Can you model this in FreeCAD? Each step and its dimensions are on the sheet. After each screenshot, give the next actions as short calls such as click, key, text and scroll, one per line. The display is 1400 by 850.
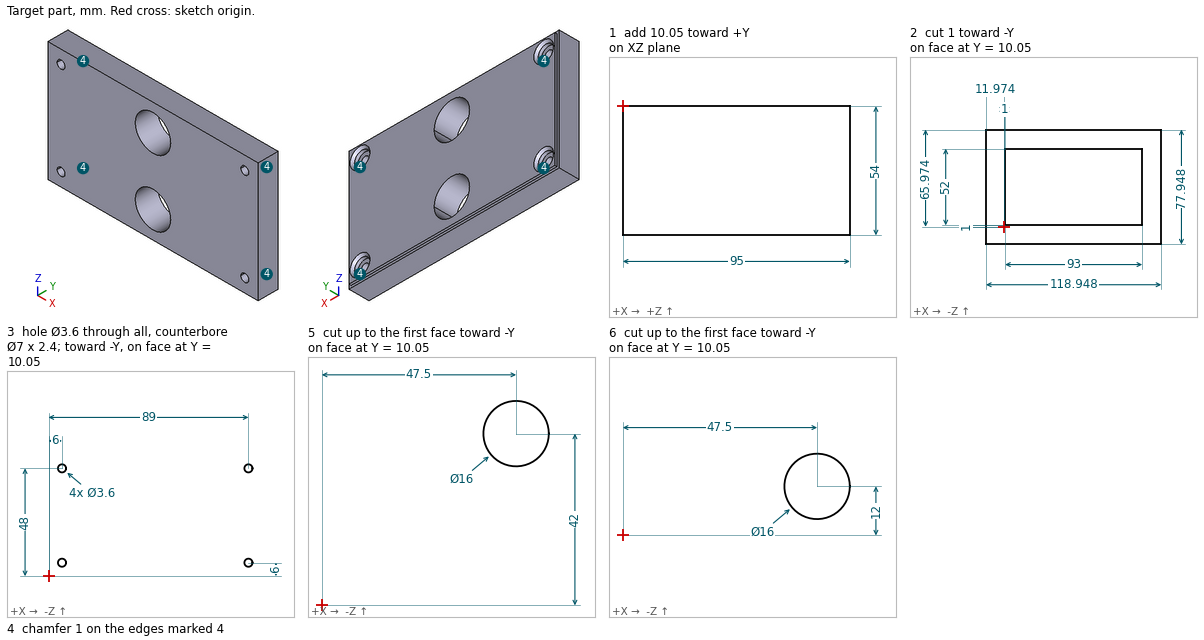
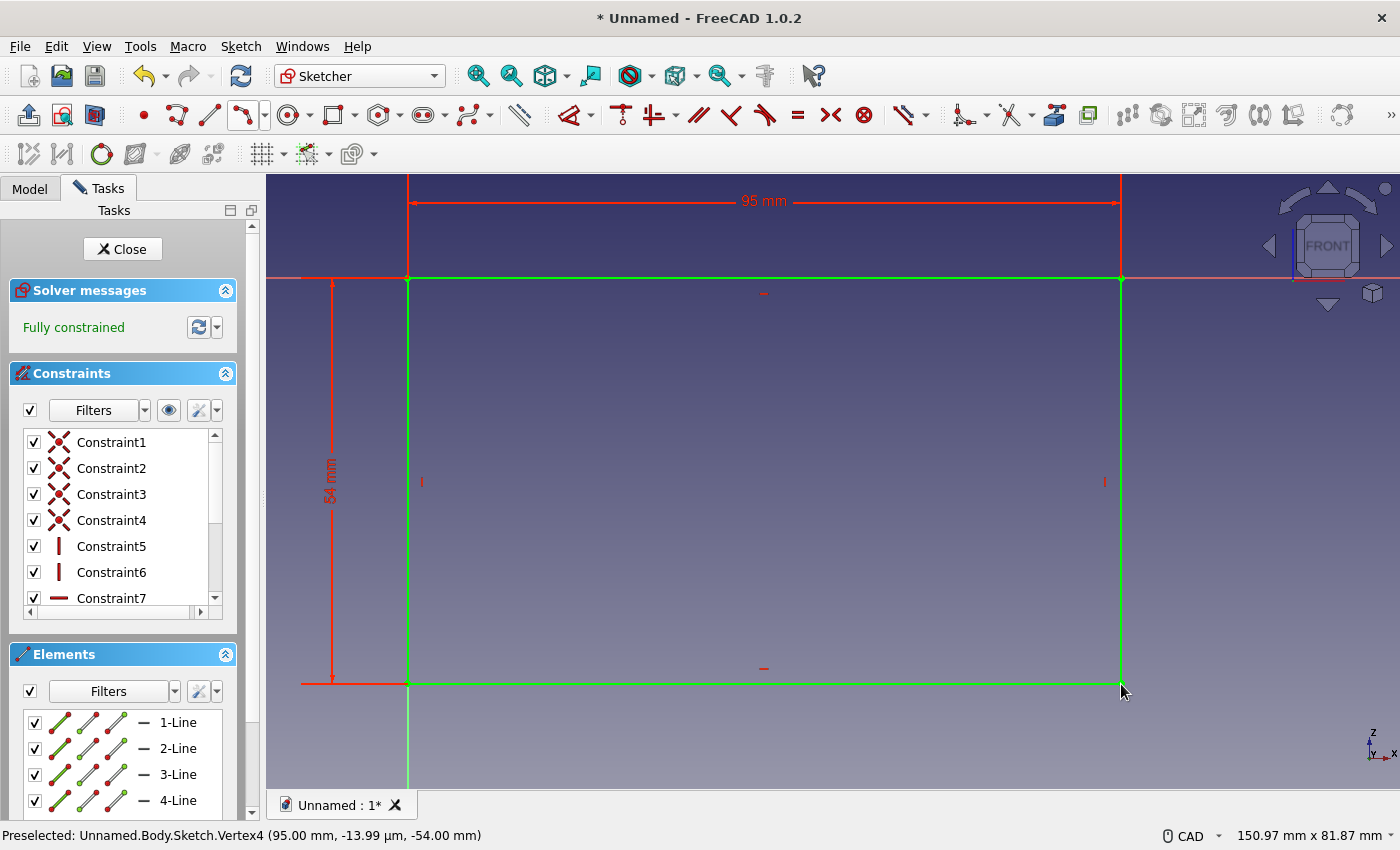
click(123, 249)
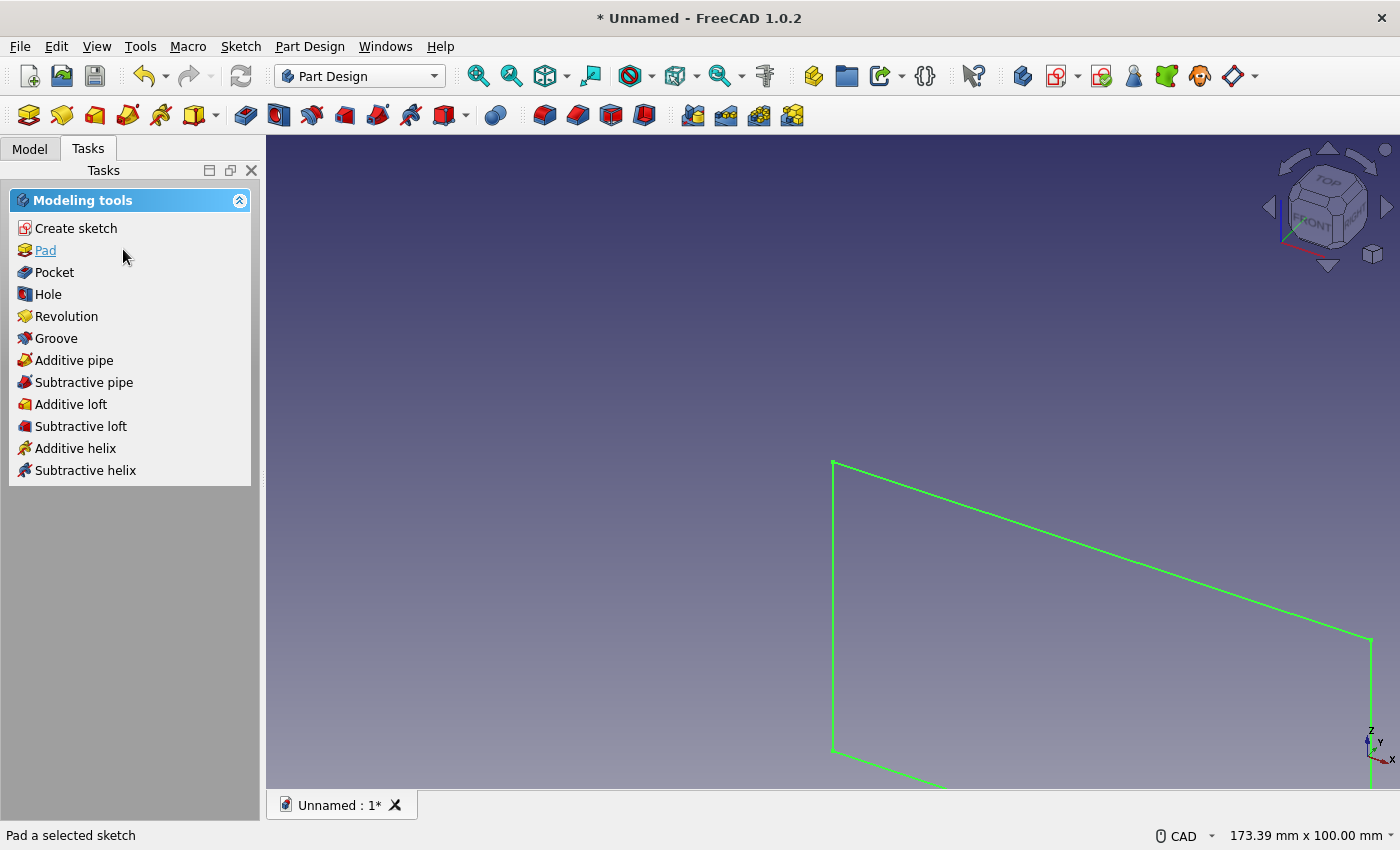
click(29, 116)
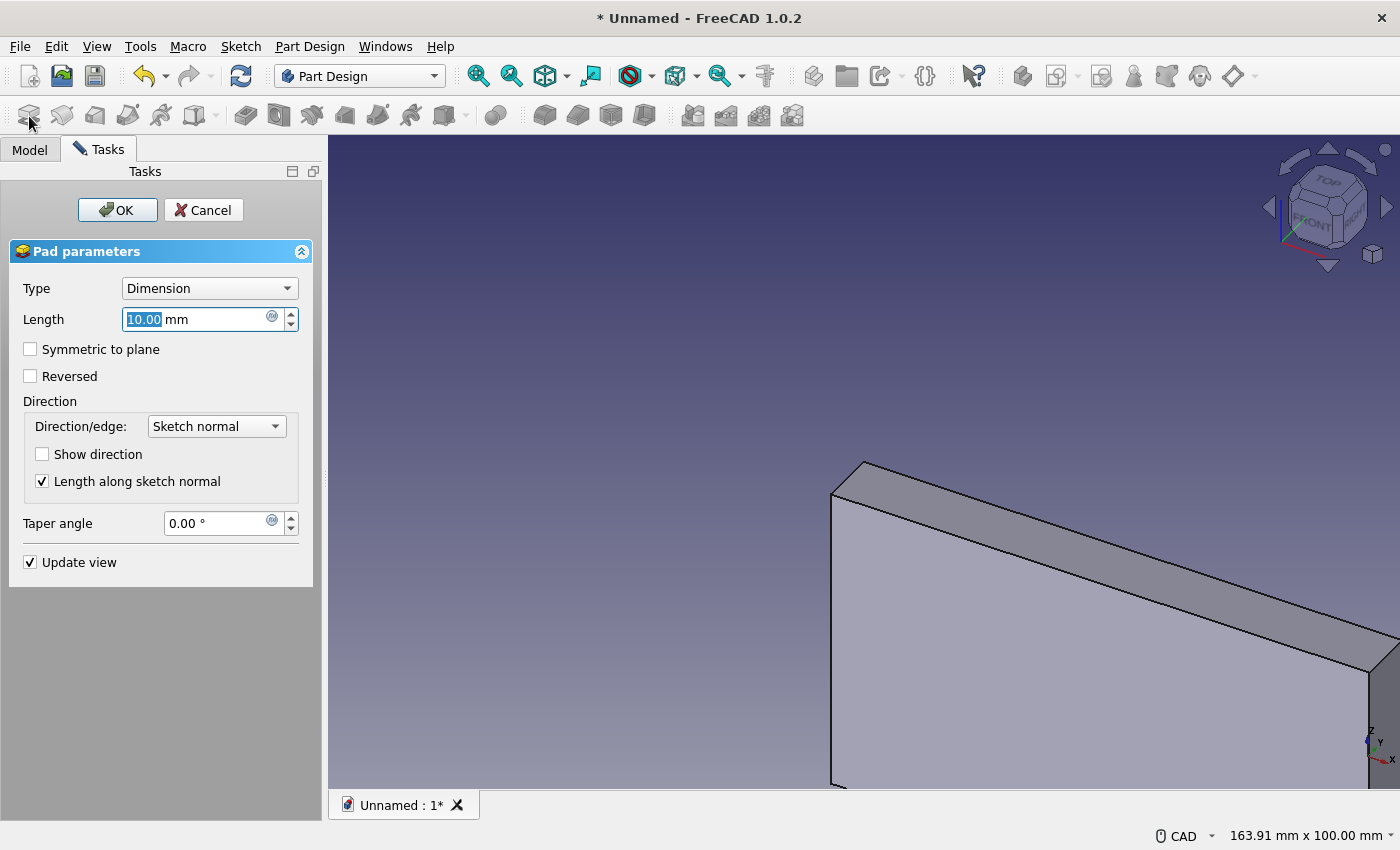
text(10.05)
key(Tab)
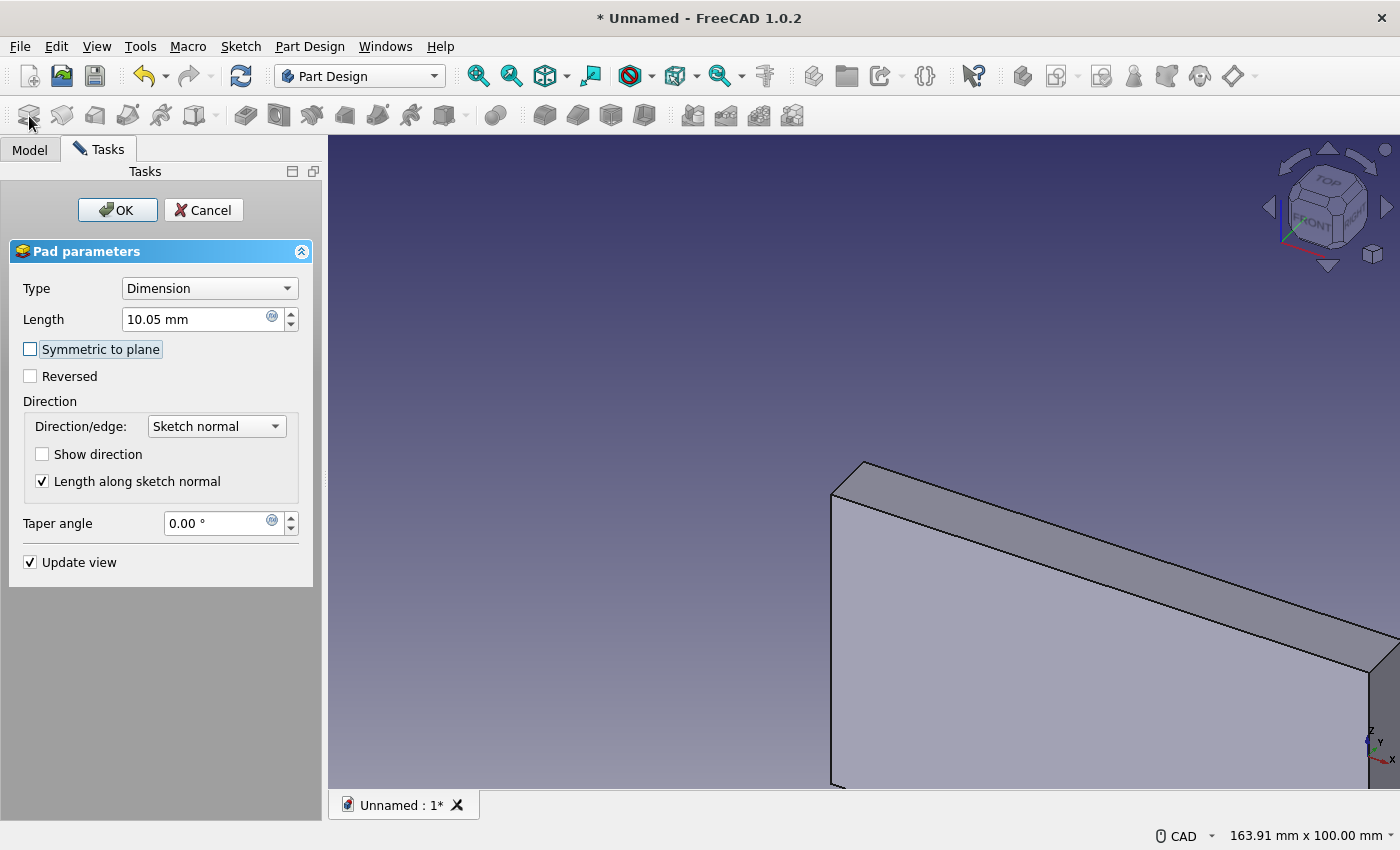
click(31, 376)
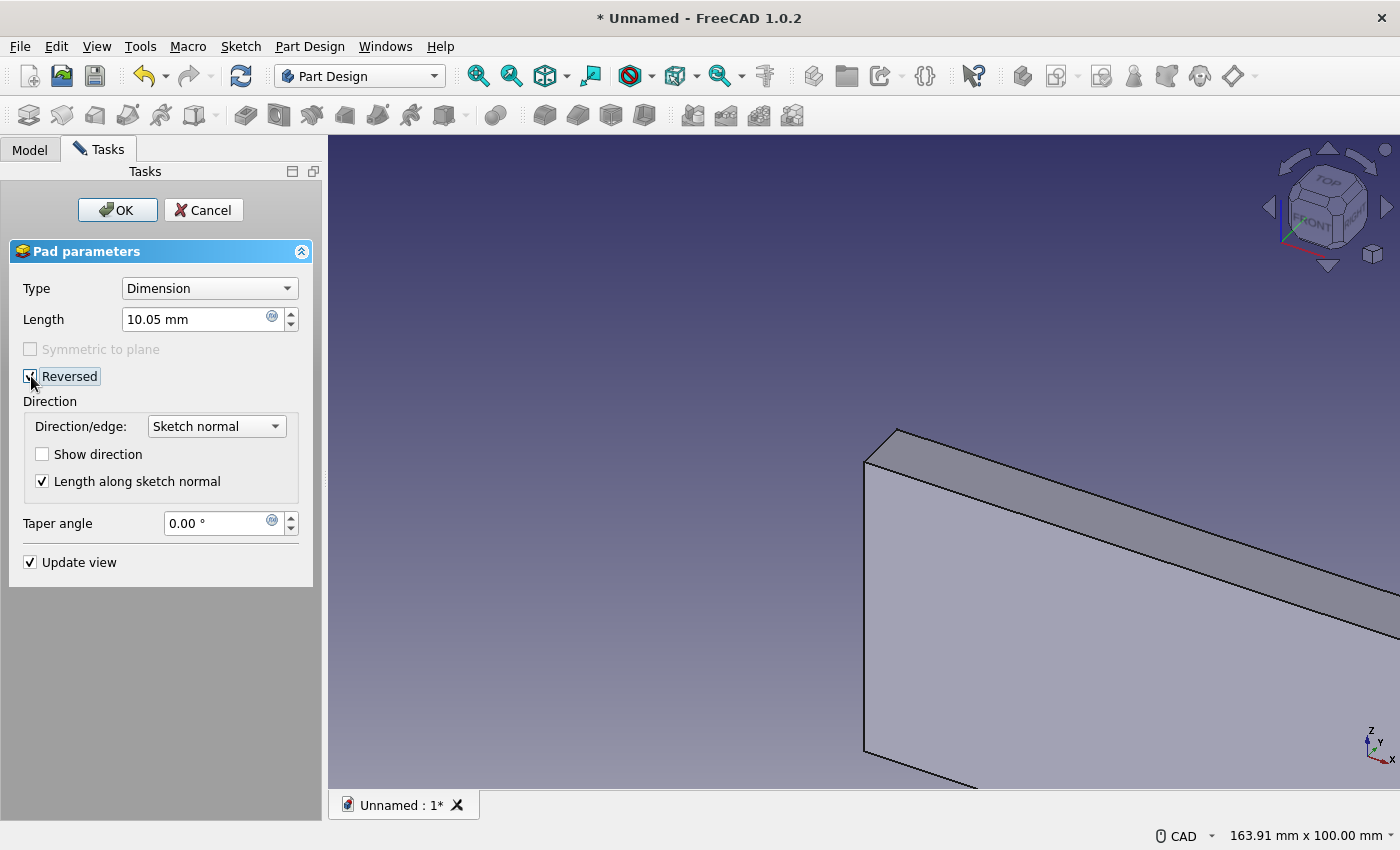
click(118, 210)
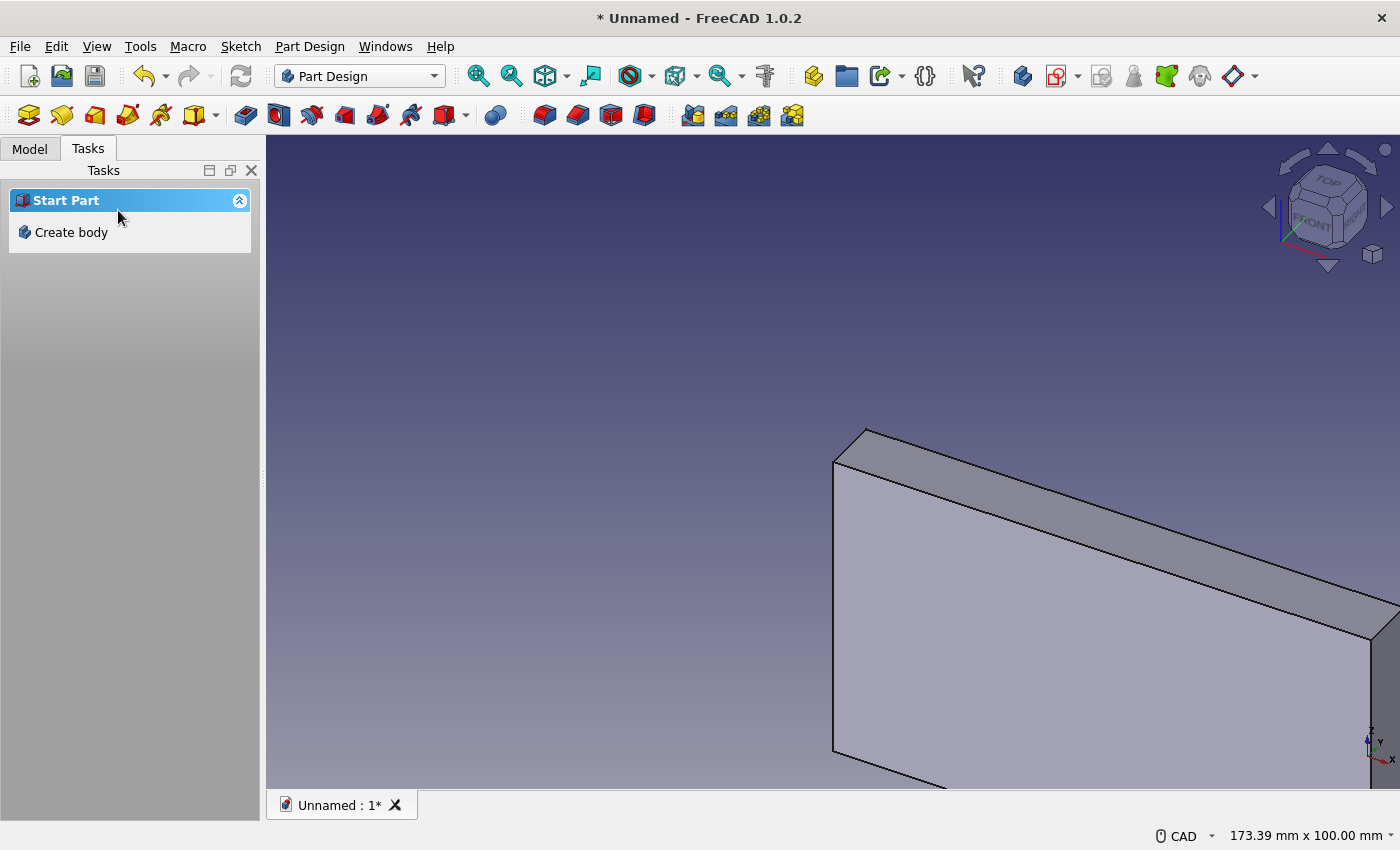
click(479, 76)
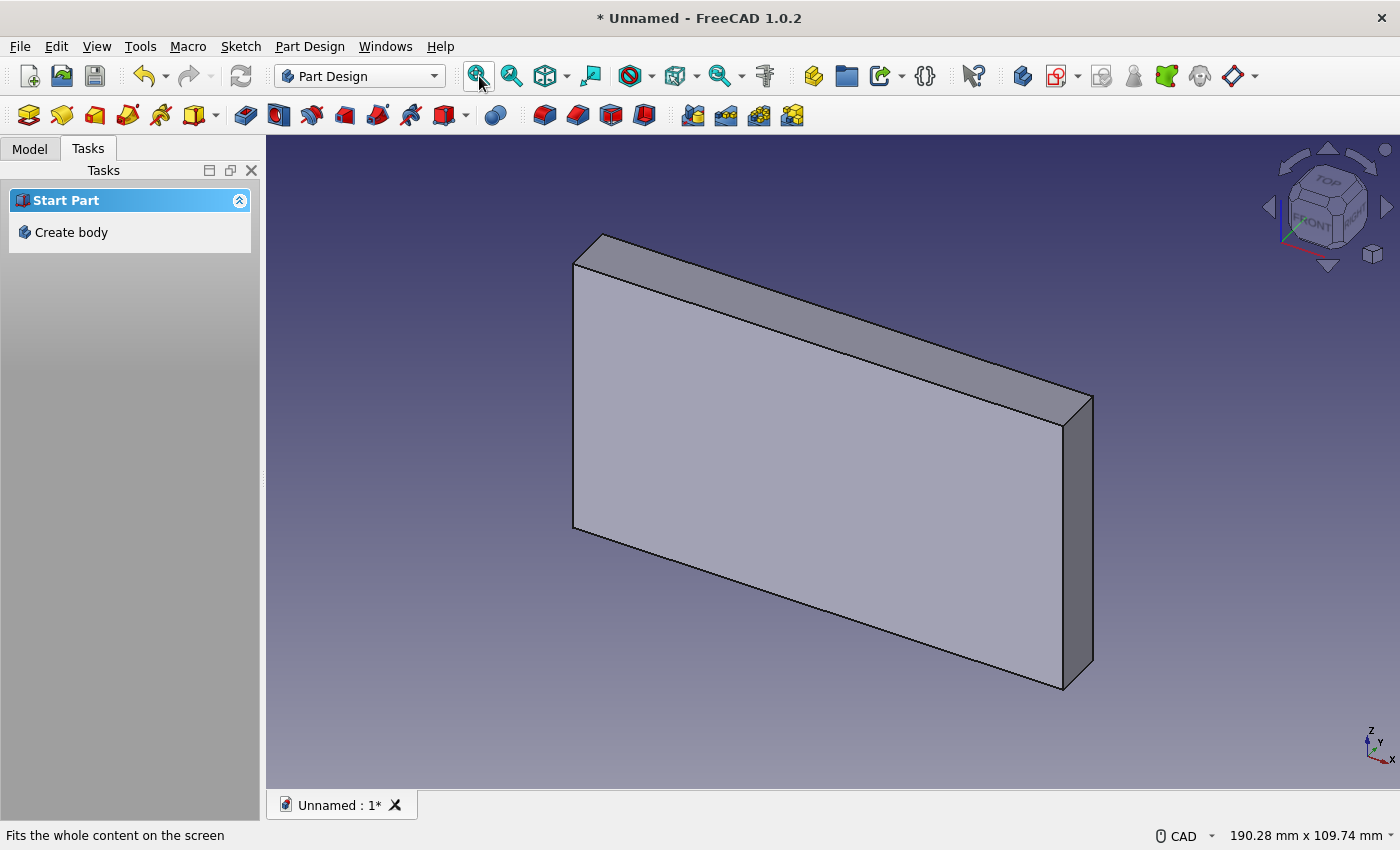
key(4)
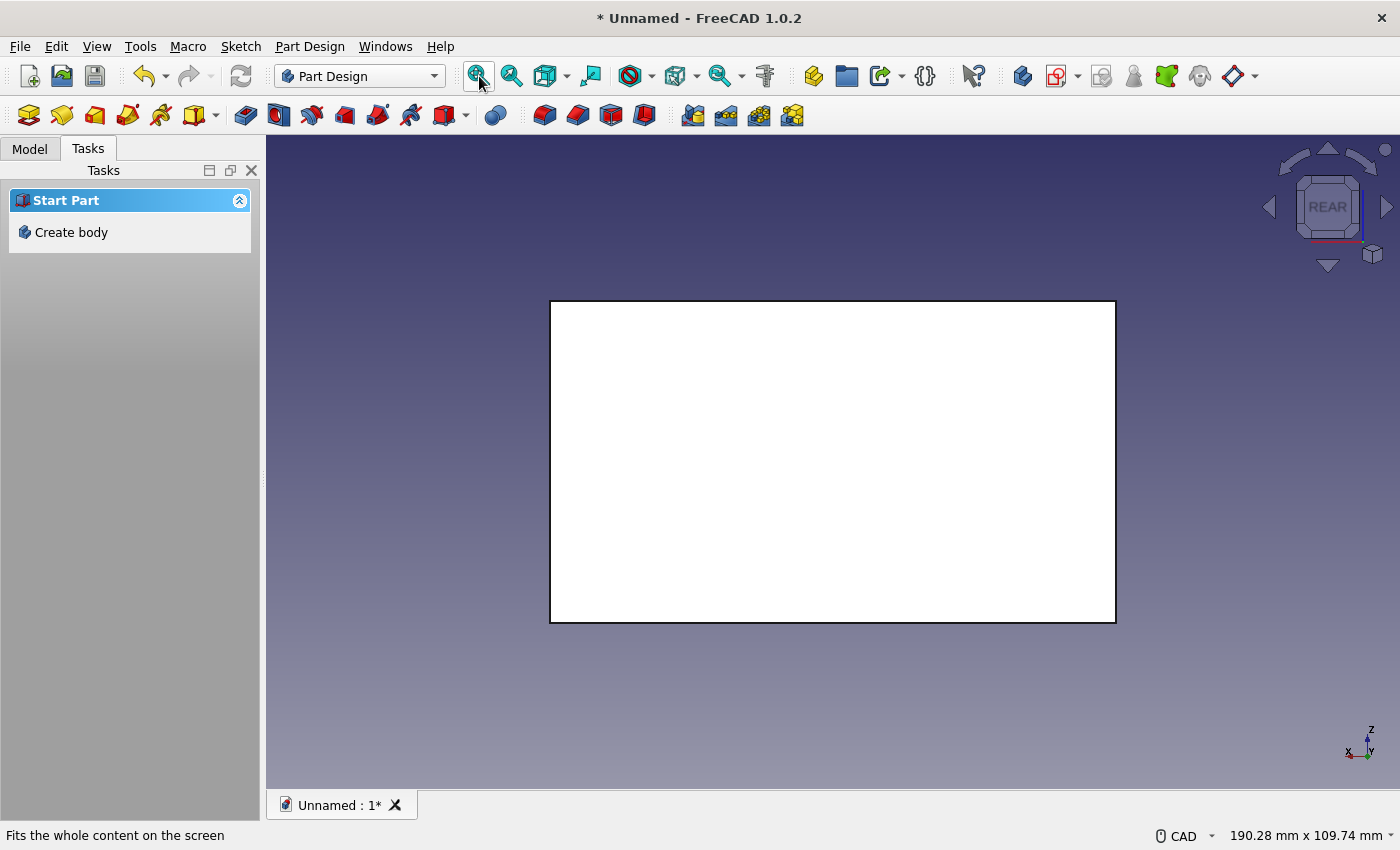
click(752, 461)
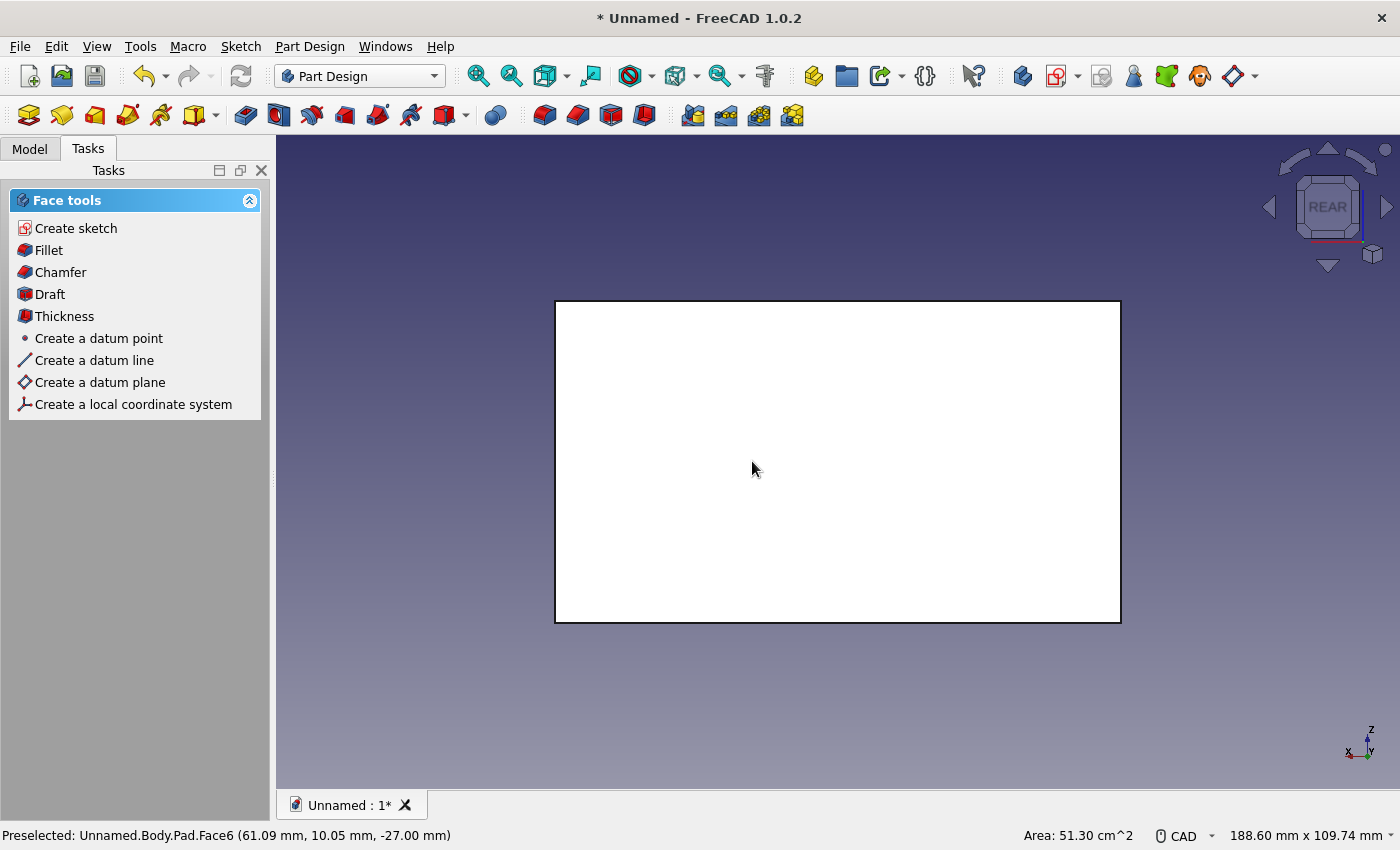
click(1056, 76)